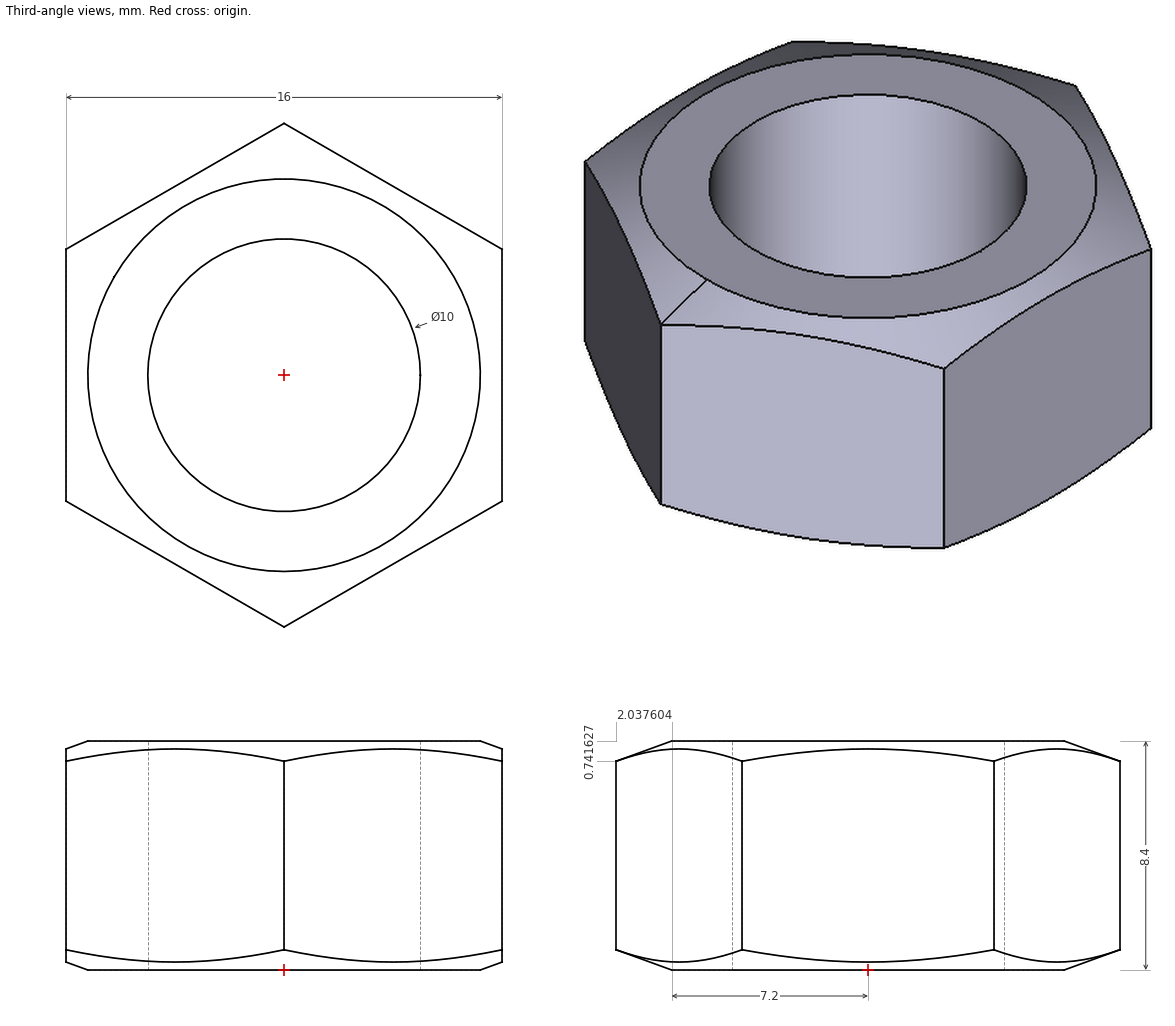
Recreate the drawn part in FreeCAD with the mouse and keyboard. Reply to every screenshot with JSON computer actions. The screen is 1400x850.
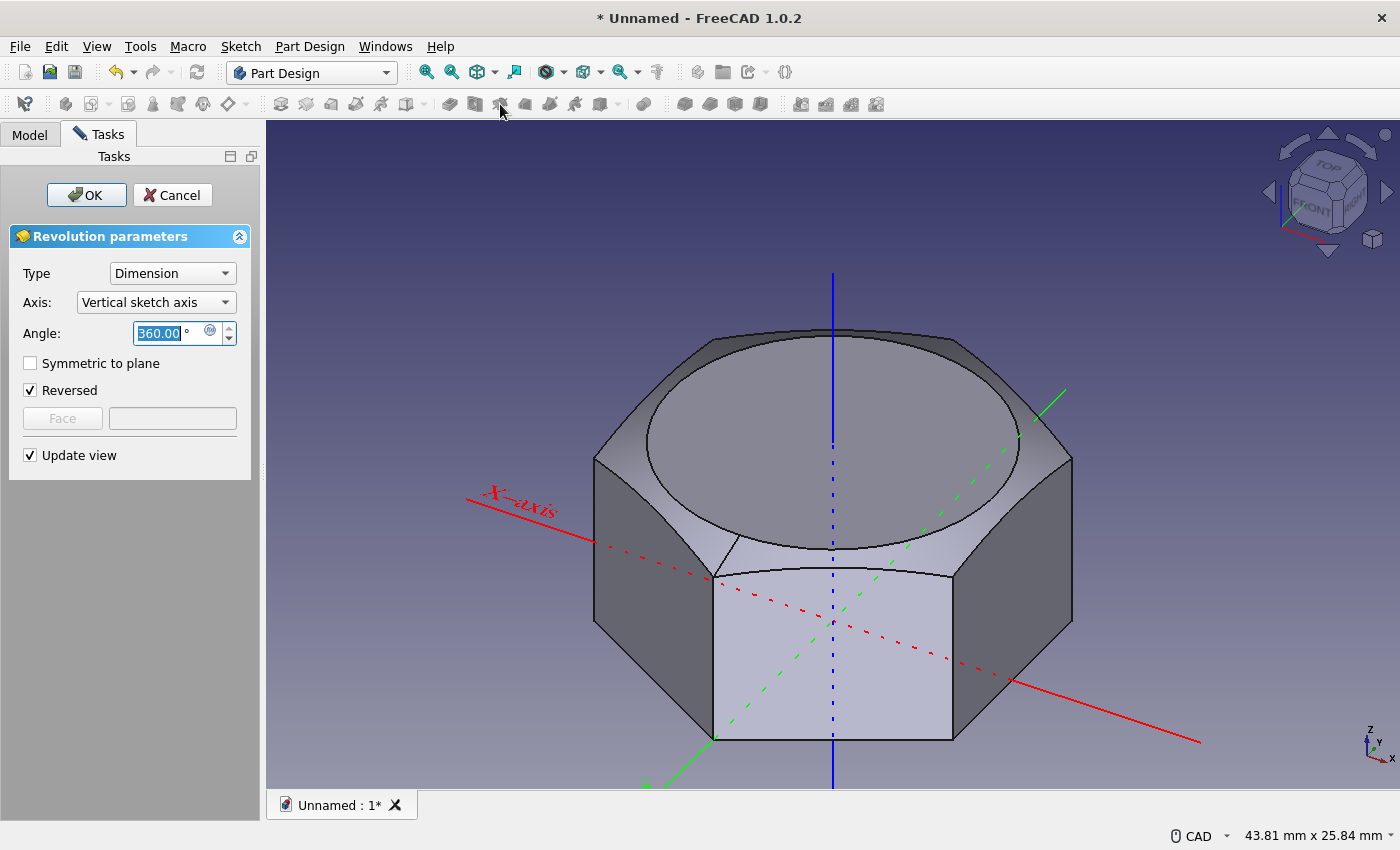
{"action": "left_click", "coordinate": [87, 195]}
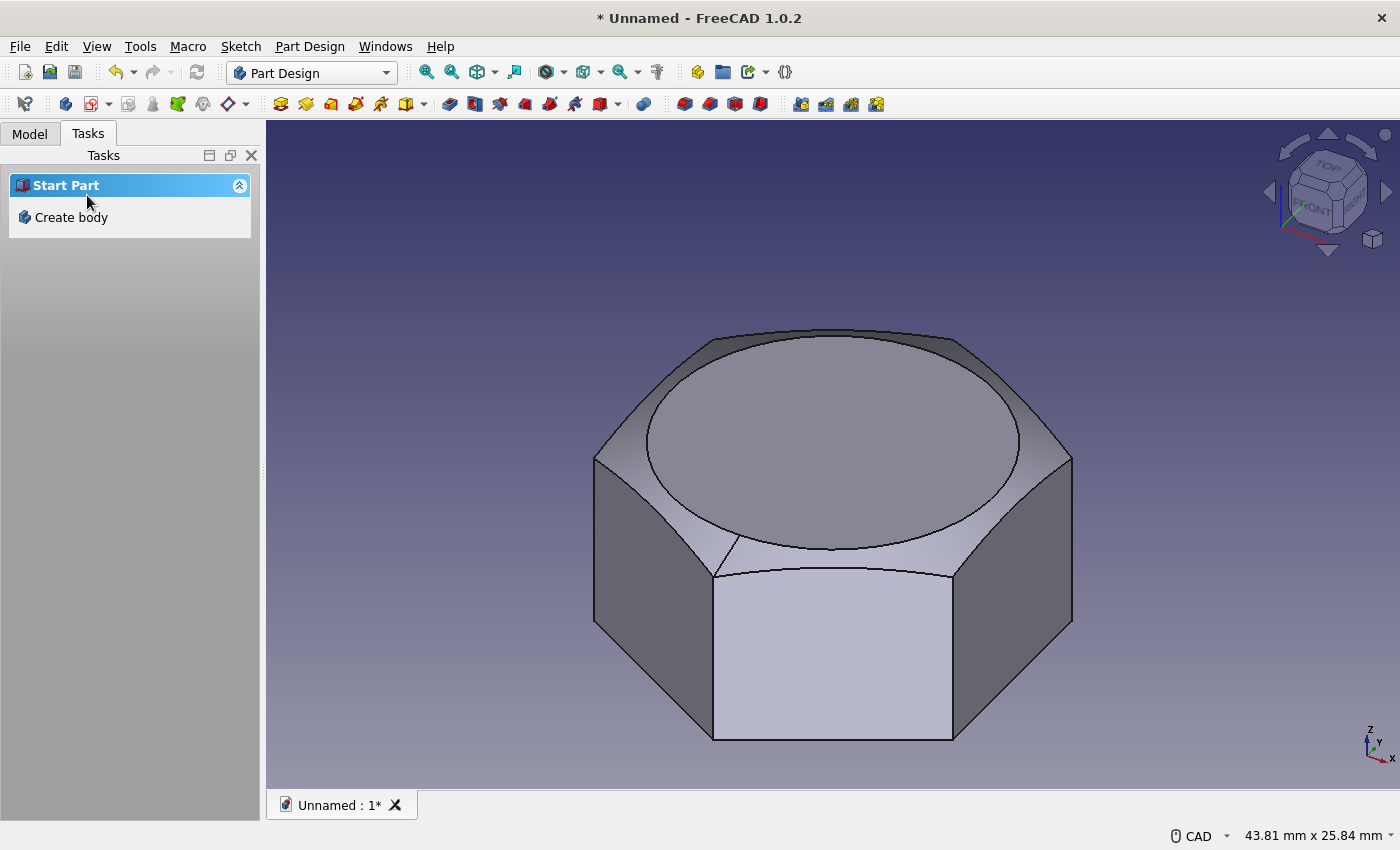
{"action": "left_click", "coordinate": [427, 72]}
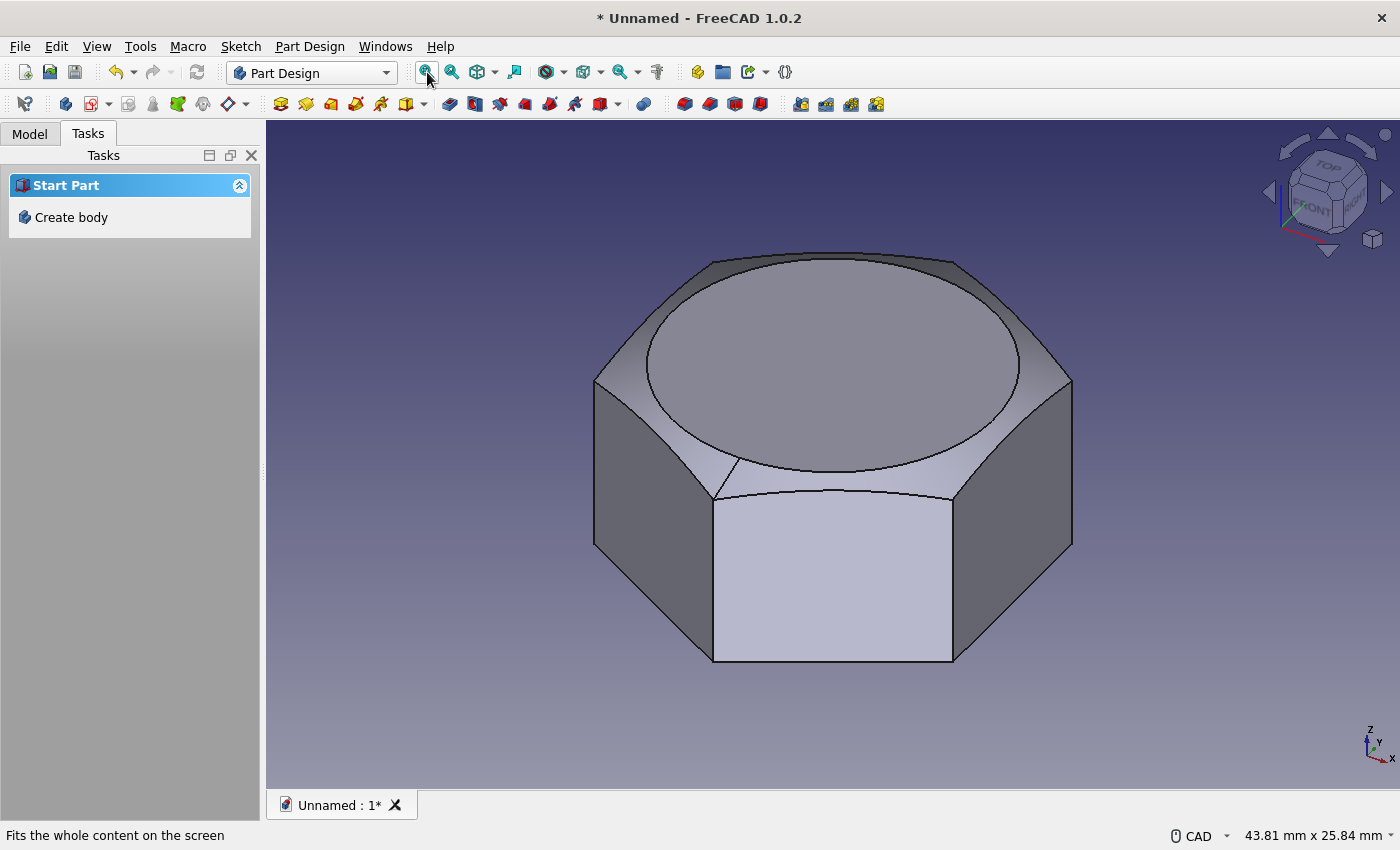
{"action": "left_click", "coordinate": [30, 134]}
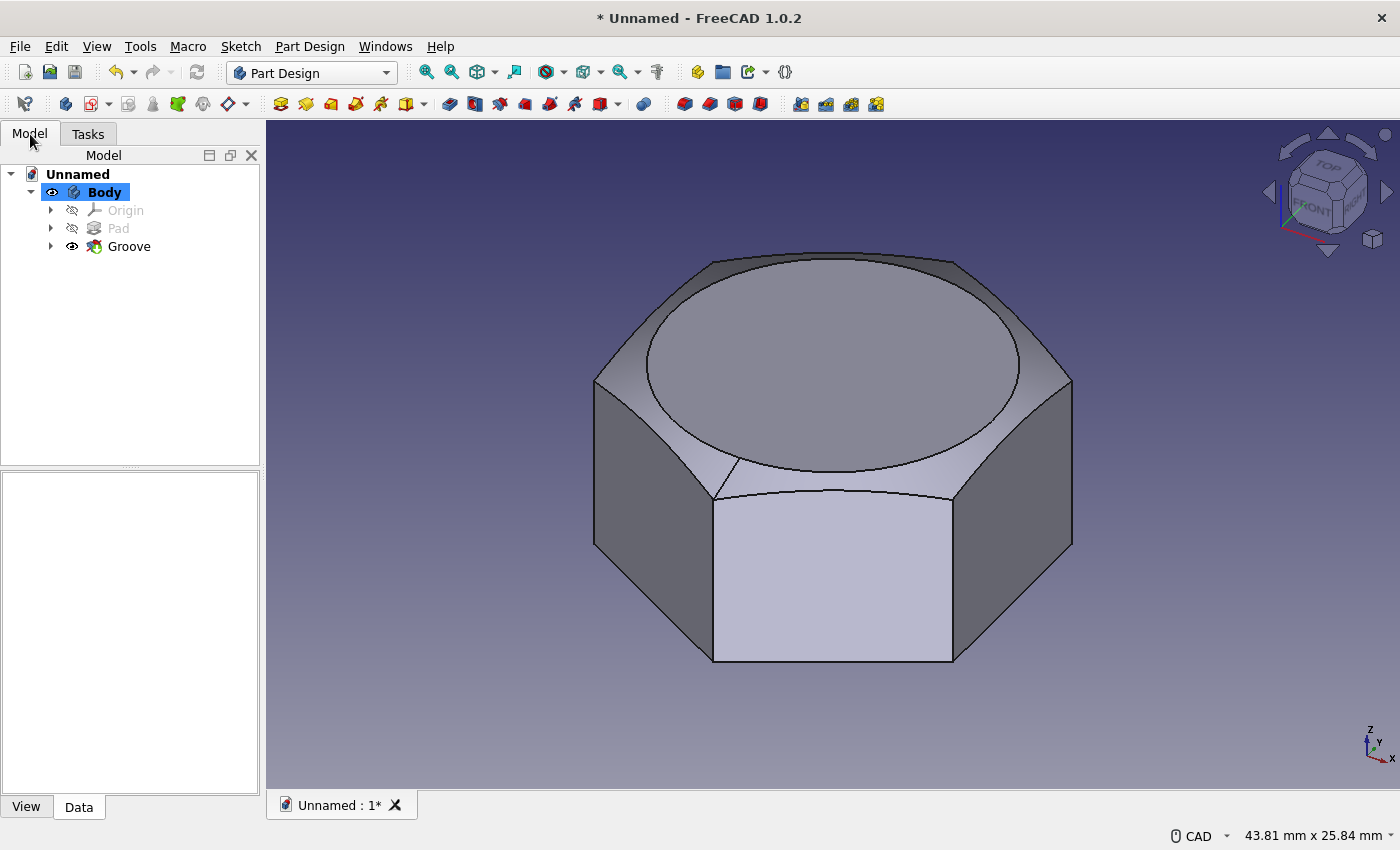
{"action": "left_click", "coordinate": [51, 210]}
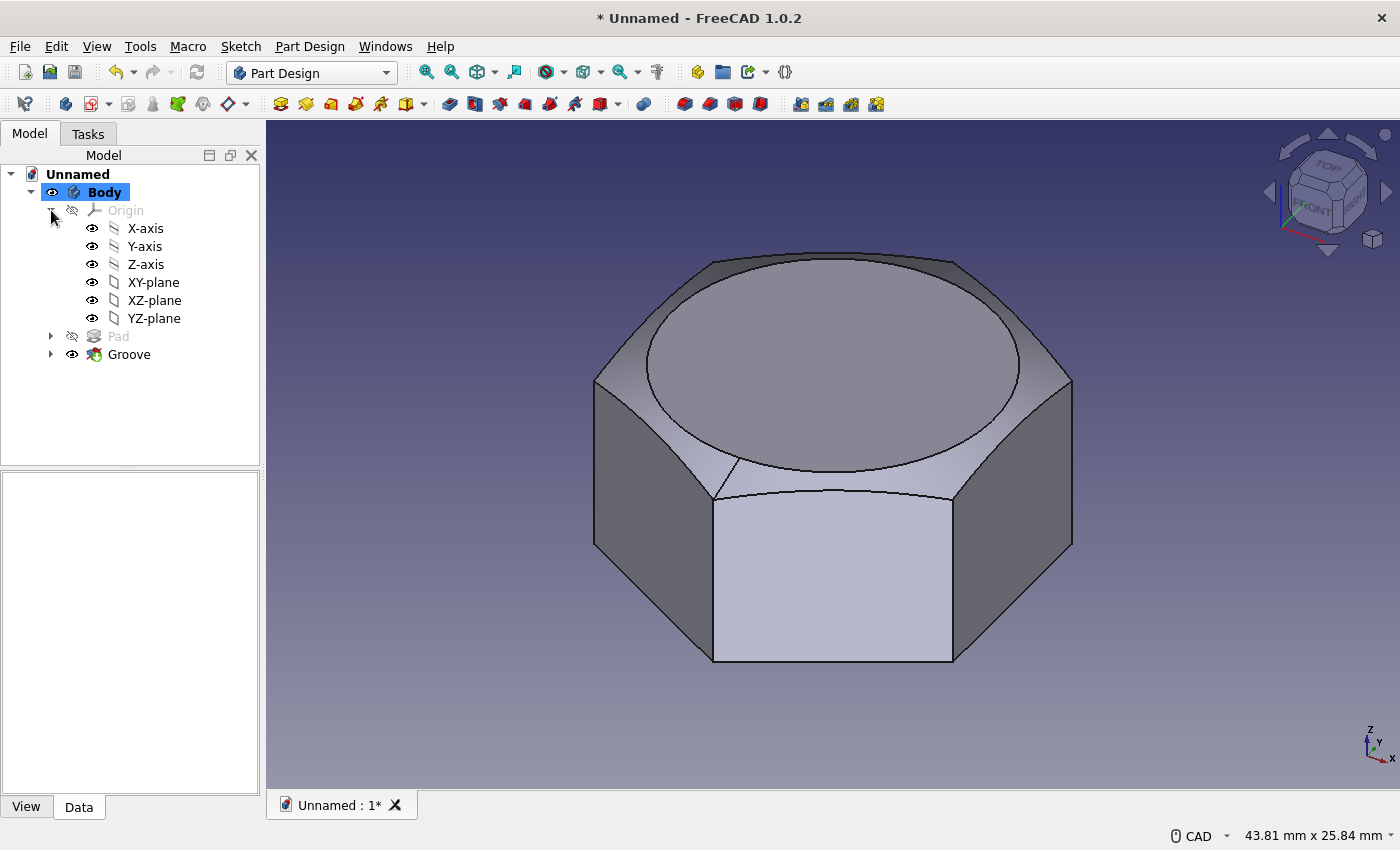
{"action": "left_click", "coordinate": [137, 282]}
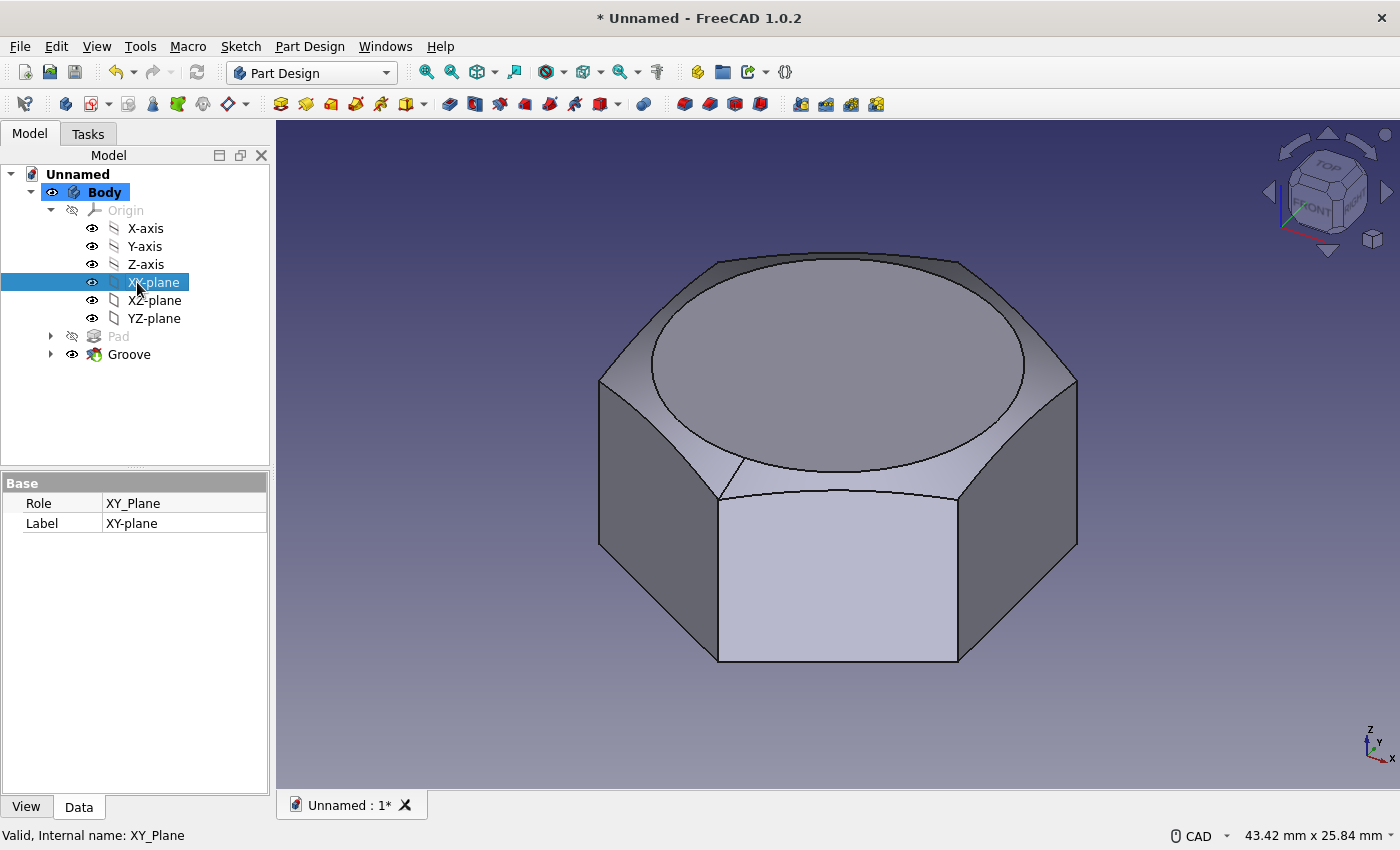
{"action": "left_click", "coordinate": [228, 104]}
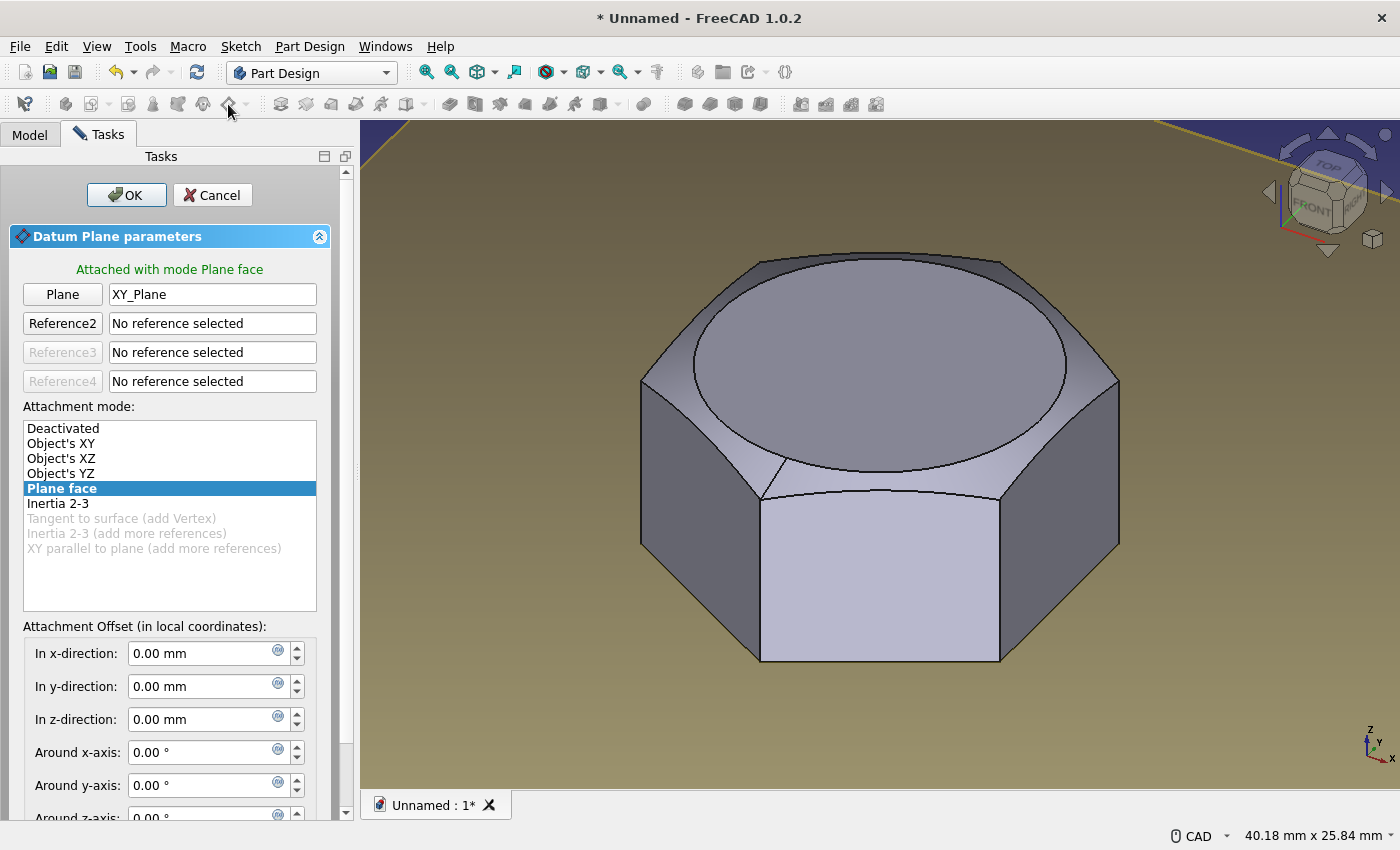
{"action": "triple_click", "coordinate": [210, 720]}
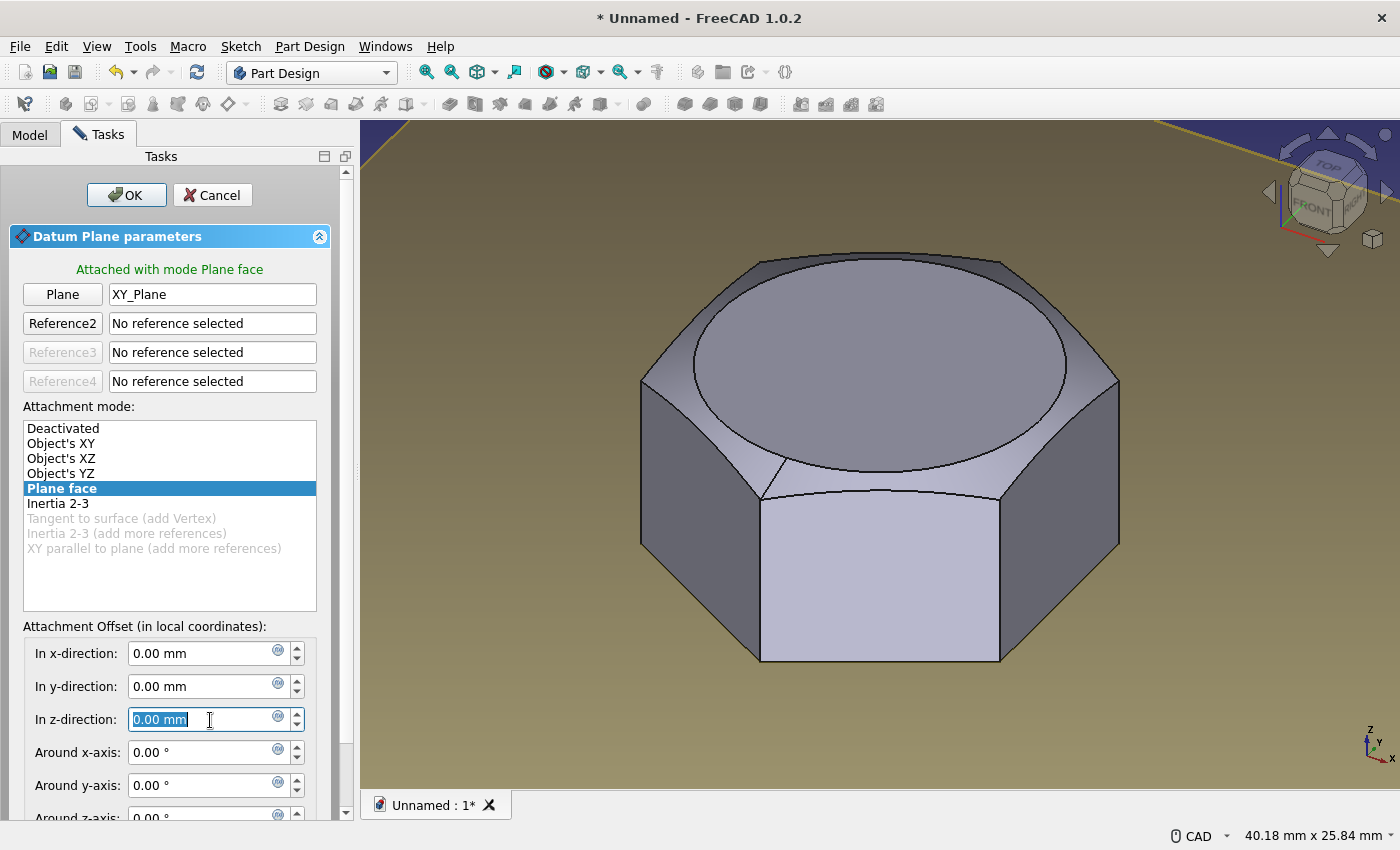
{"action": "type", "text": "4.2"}
{"action": "key", "text": "Tab"}